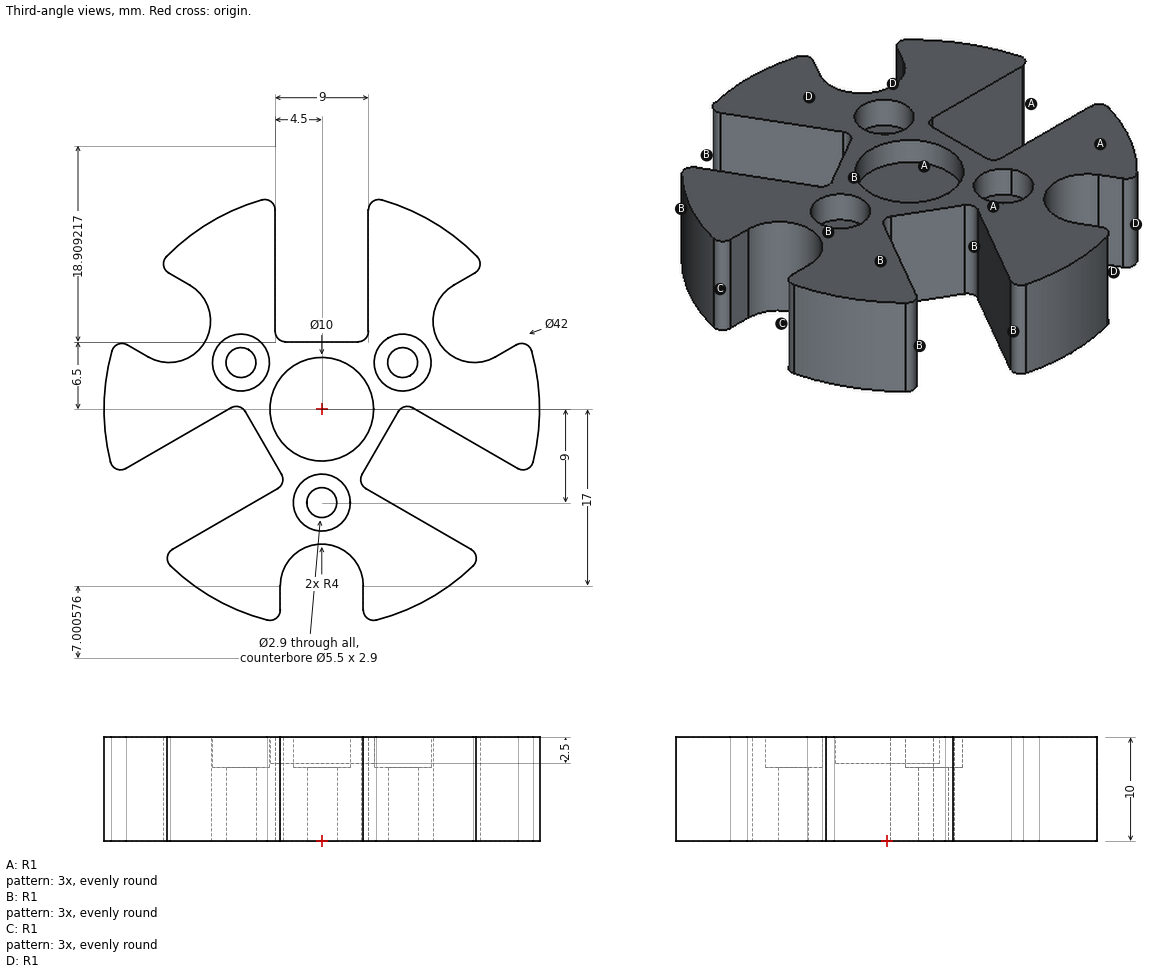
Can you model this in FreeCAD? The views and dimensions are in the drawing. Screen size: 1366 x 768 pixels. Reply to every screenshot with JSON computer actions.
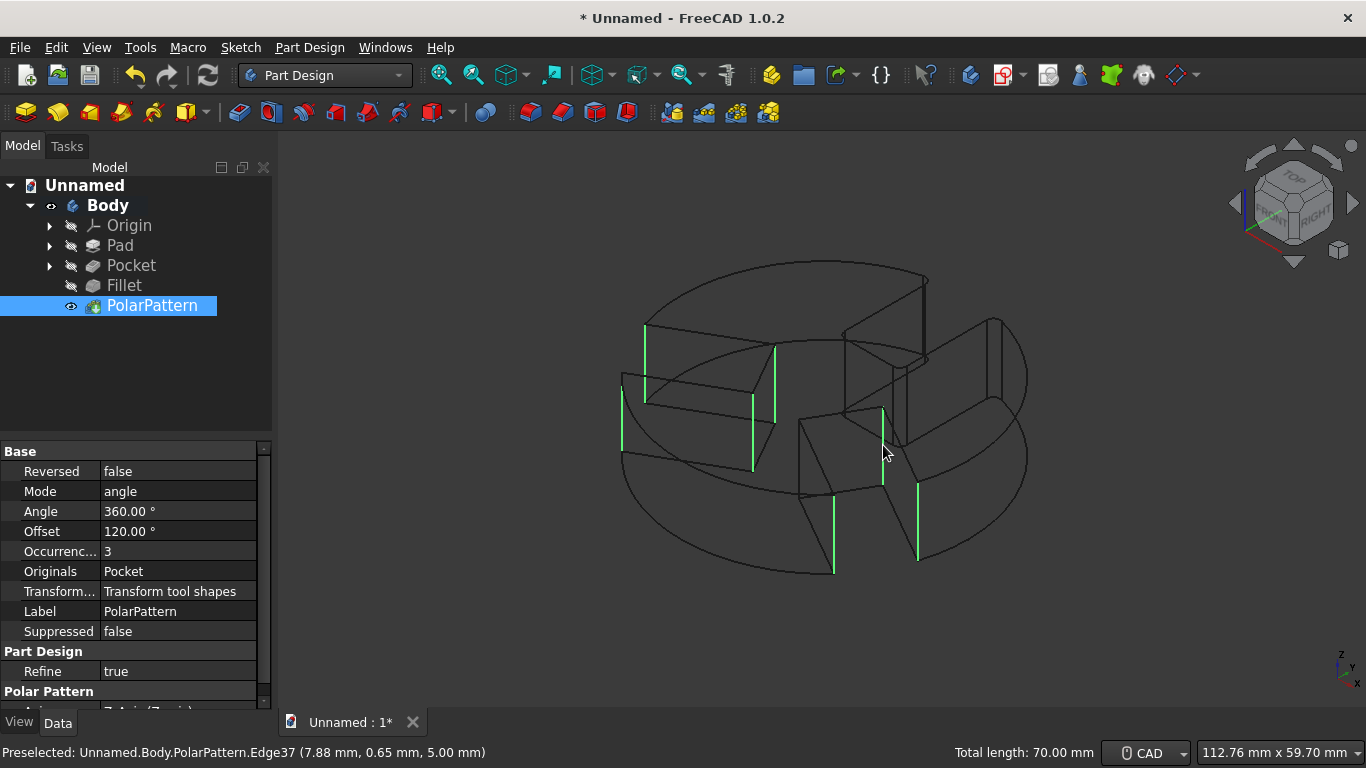
{"action": "left_click", "coordinate": [799, 458], "text": "ctrl"}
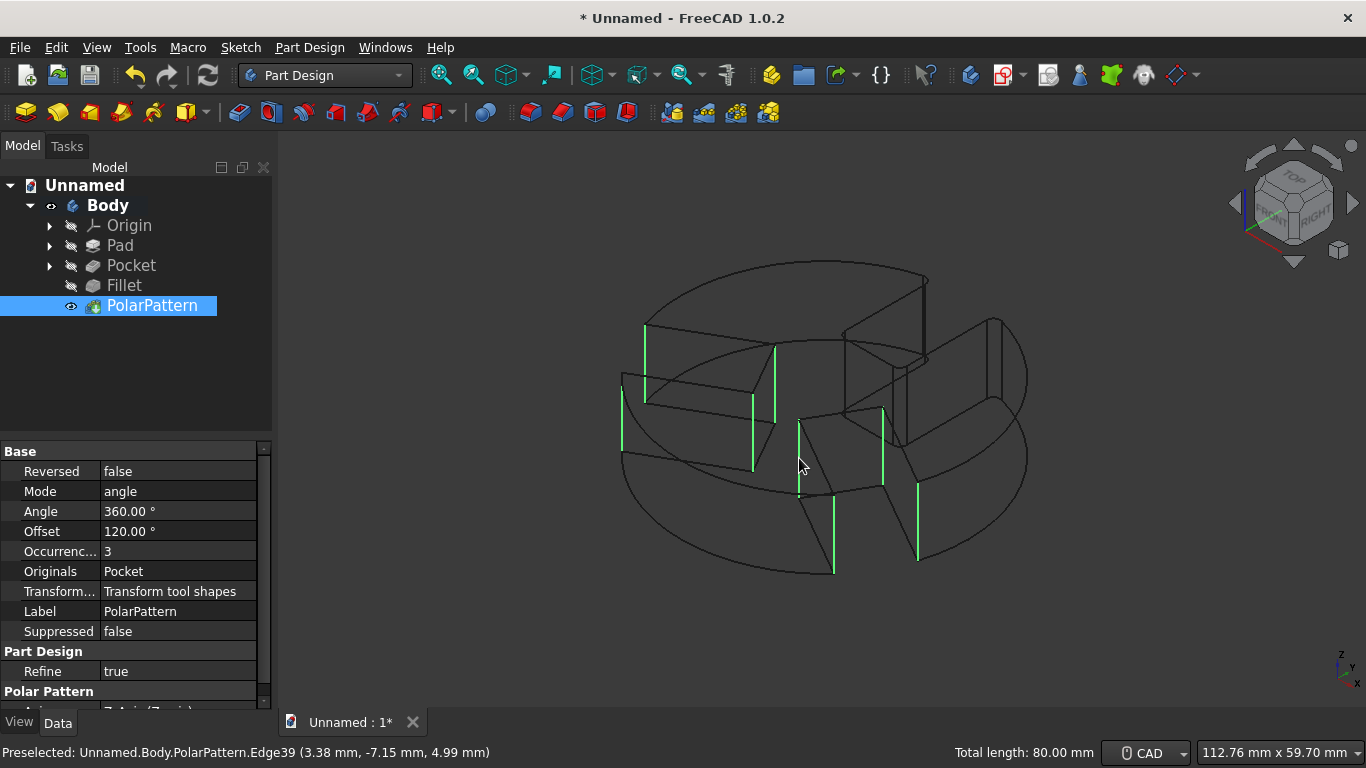
{"action": "key", "text": "v 1"}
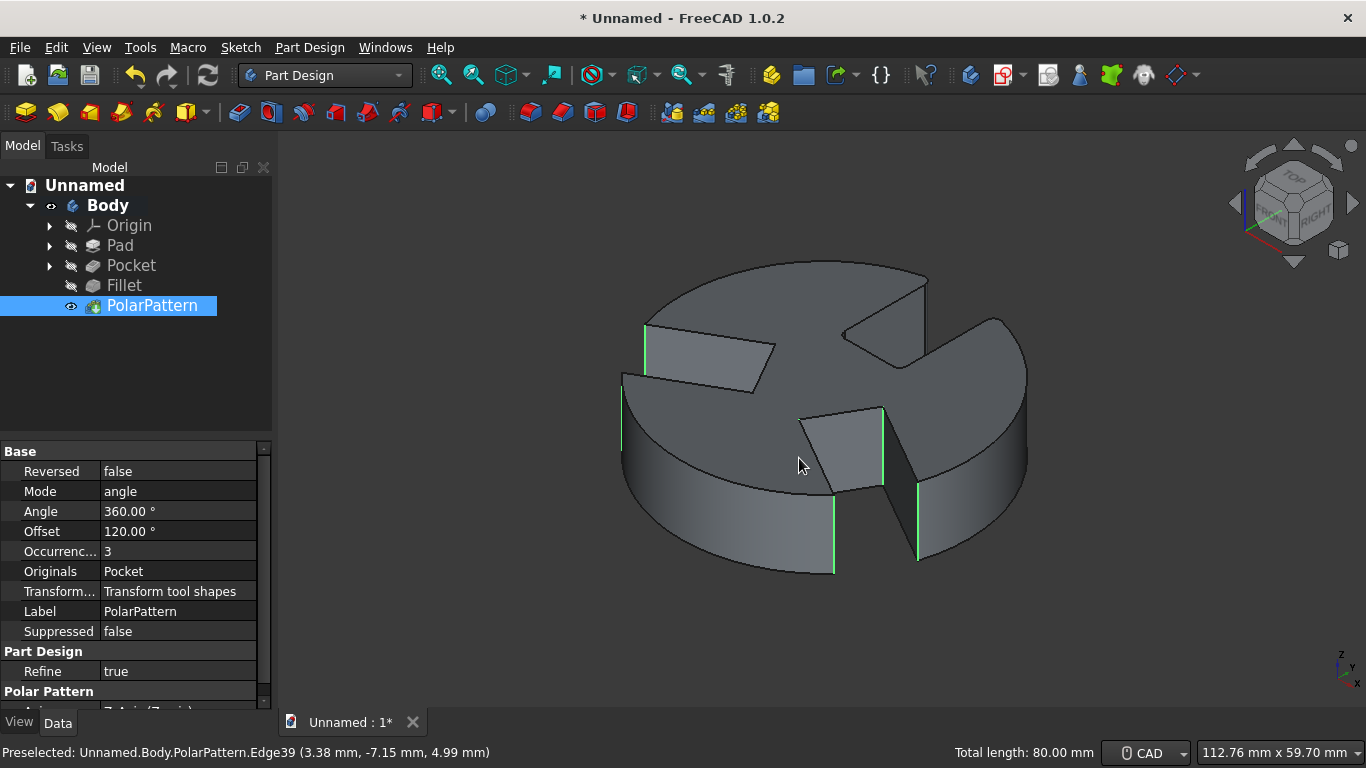
{"action": "left_click", "coordinate": [532, 112]}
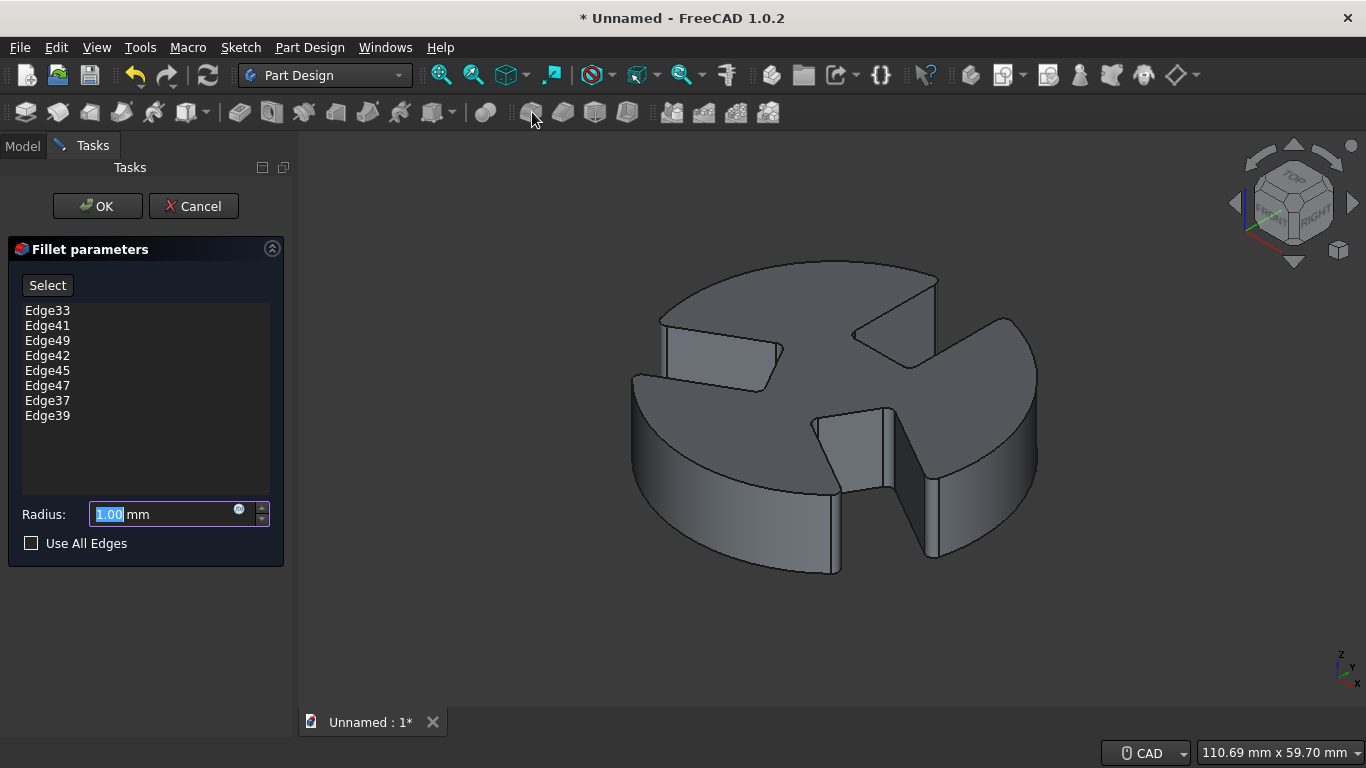
{"action": "type", "text": "1"}
{"action": "key", "text": "Tab"}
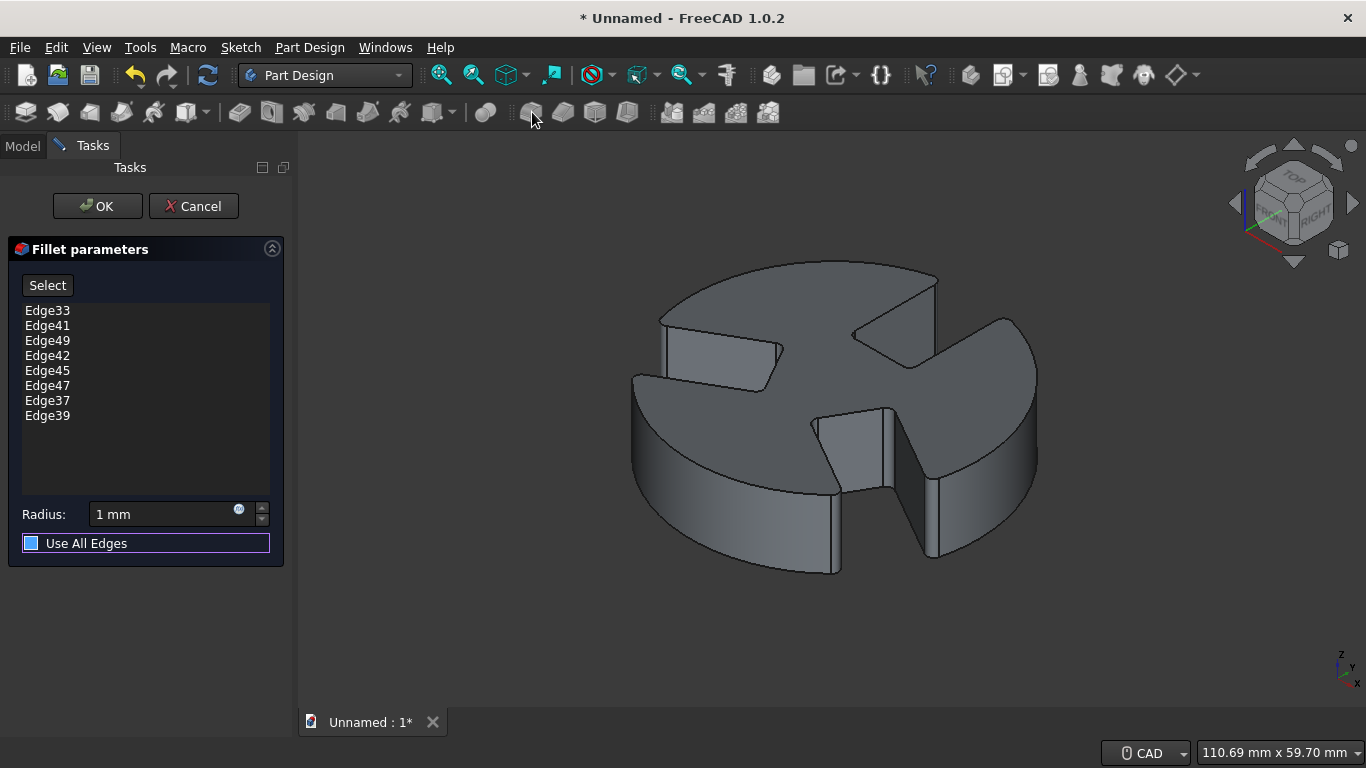
{"action": "left_click", "coordinate": [98, 206]}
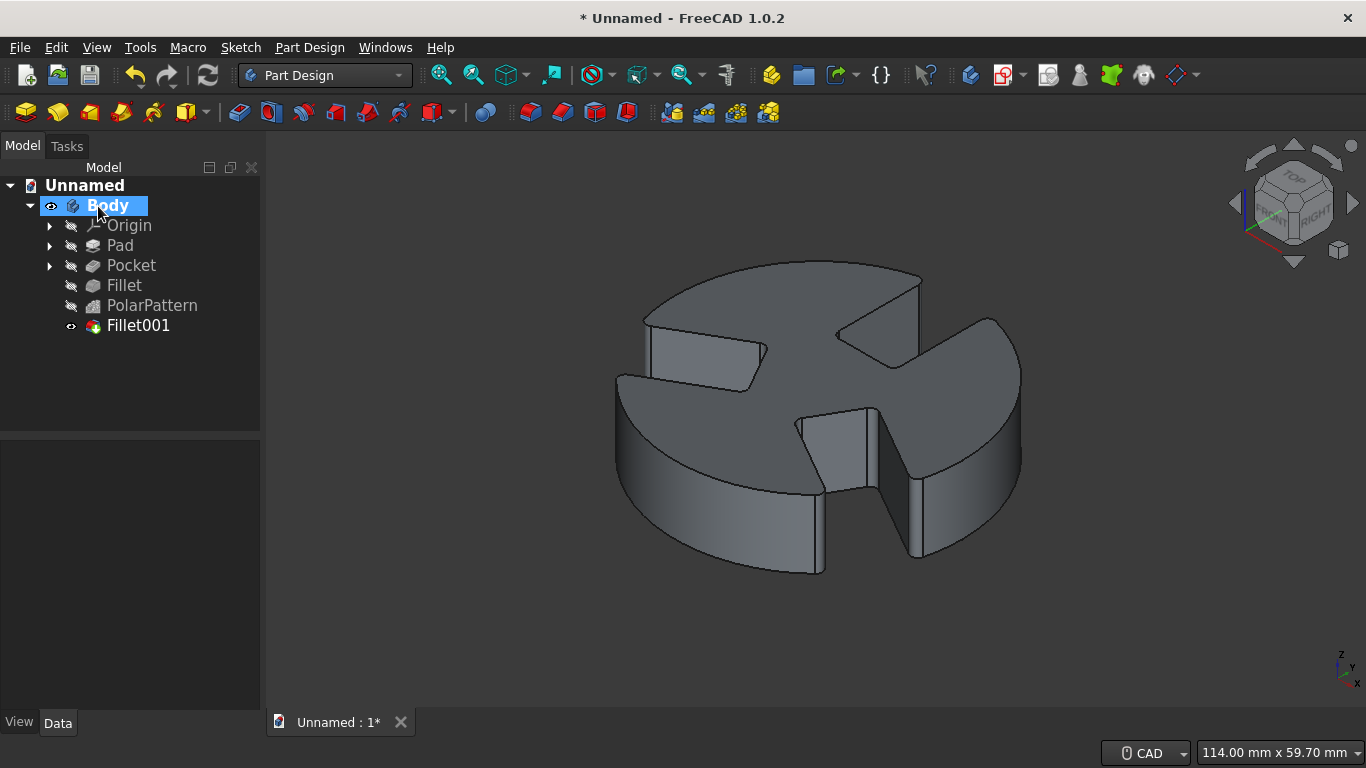
{"action": "left_click", "coordinate": [816, 379]}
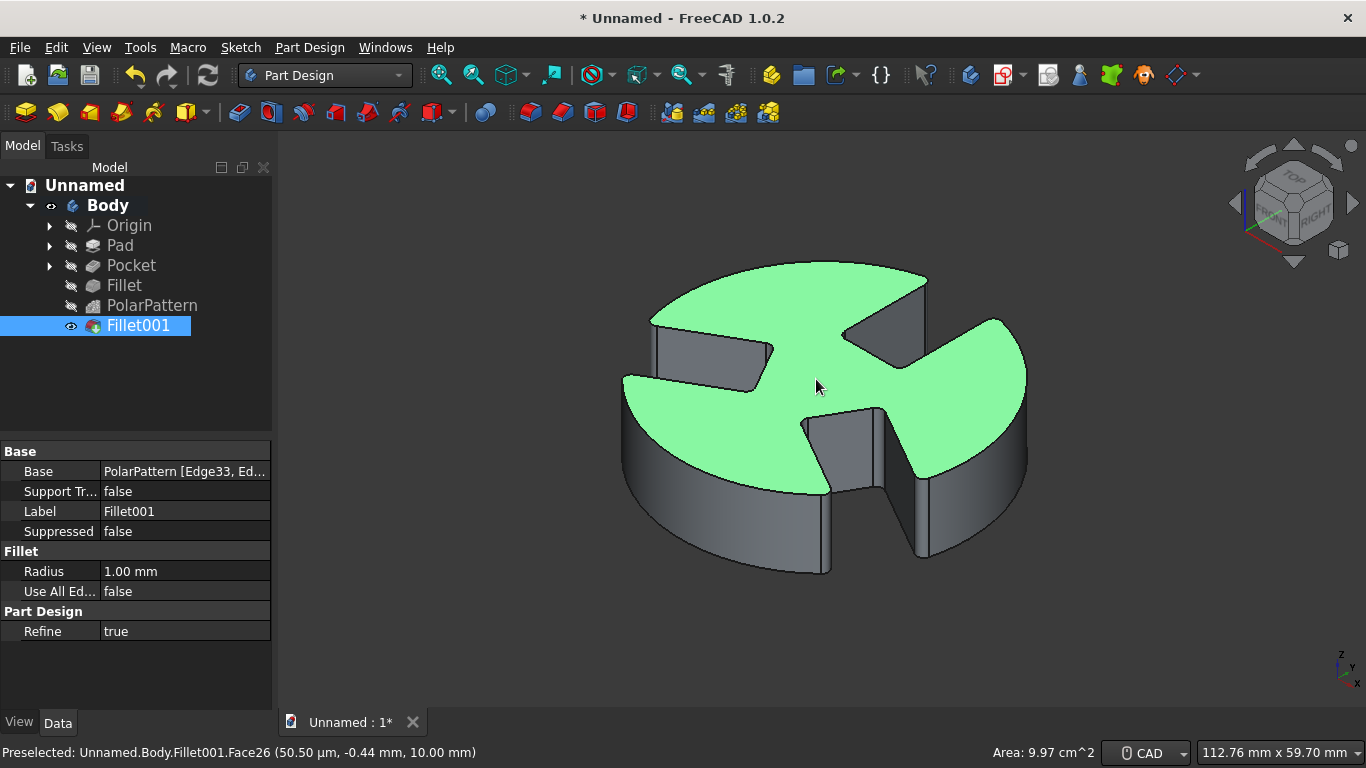
{"action": "left_click", "coordinate": [1004, 76]}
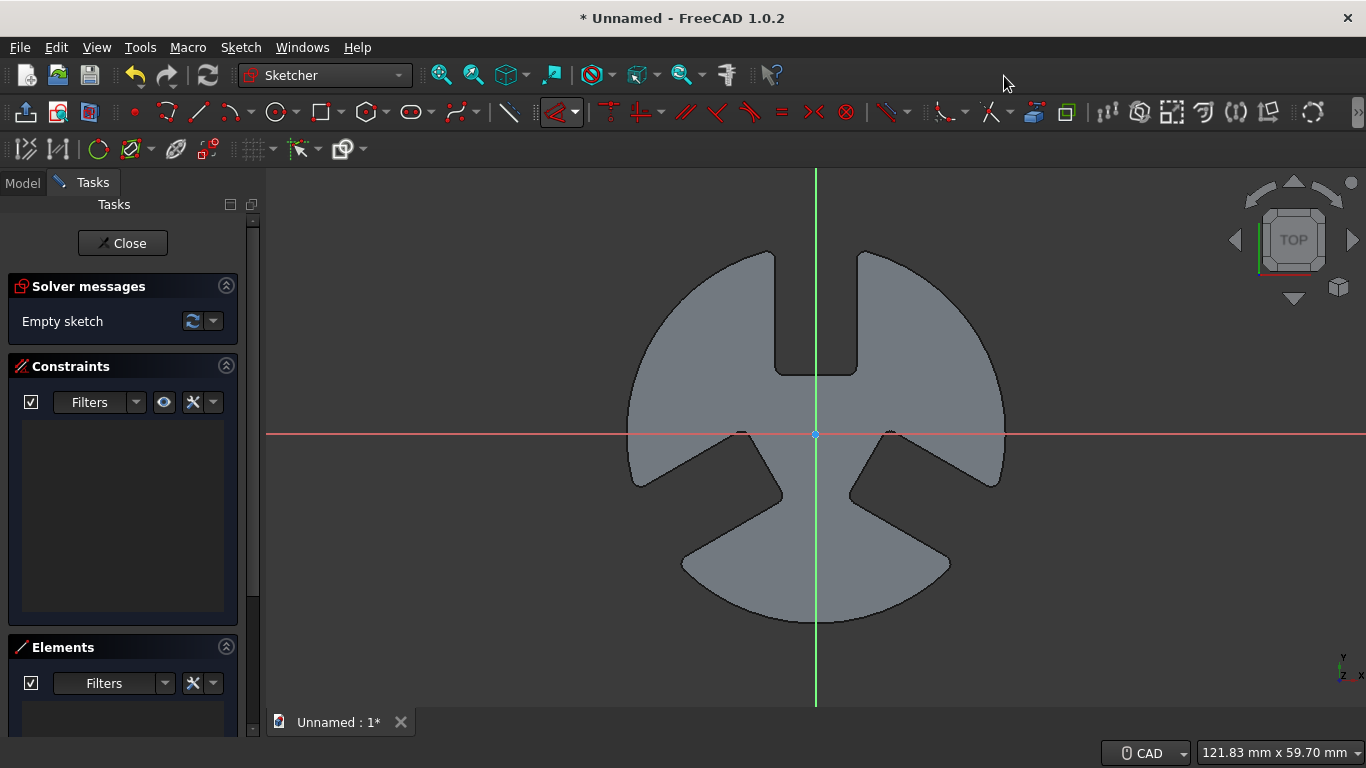
{"action": "scroll", "coordinate": [821, 522], "scroll_direction": "up", "scroll_amount": 13}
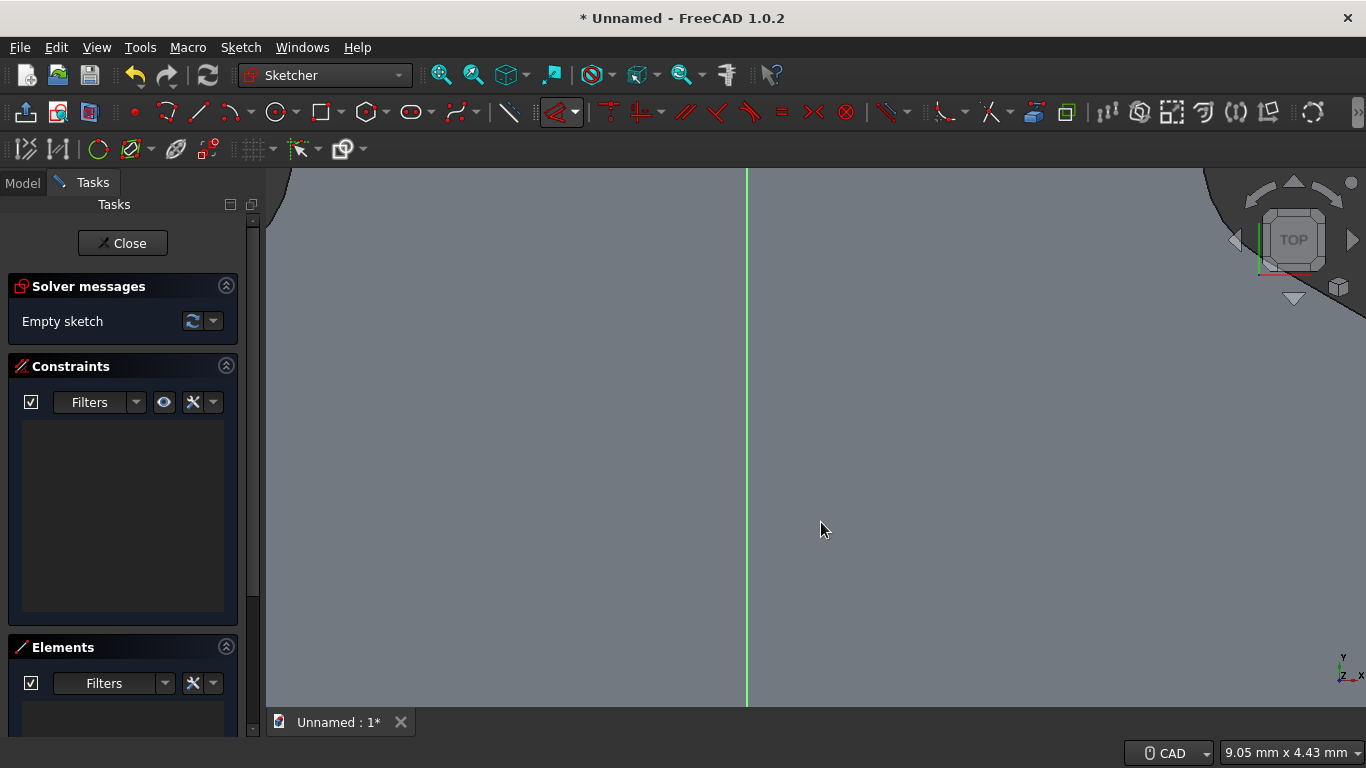
{"action": "left_click", "coordinate": [276, 112]}